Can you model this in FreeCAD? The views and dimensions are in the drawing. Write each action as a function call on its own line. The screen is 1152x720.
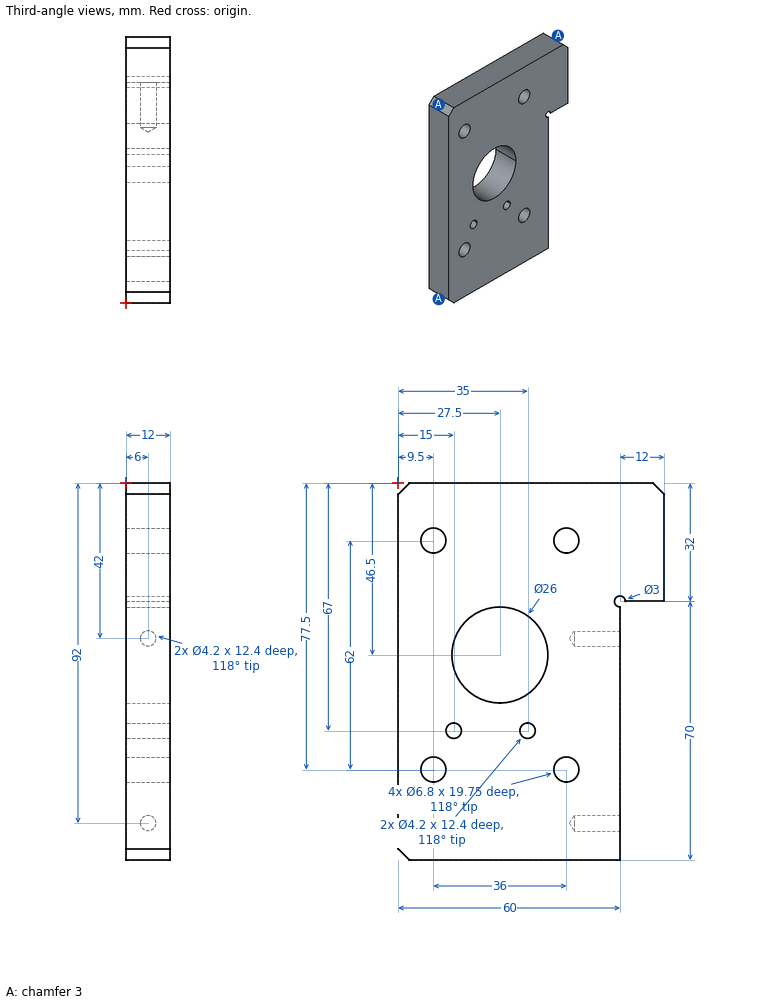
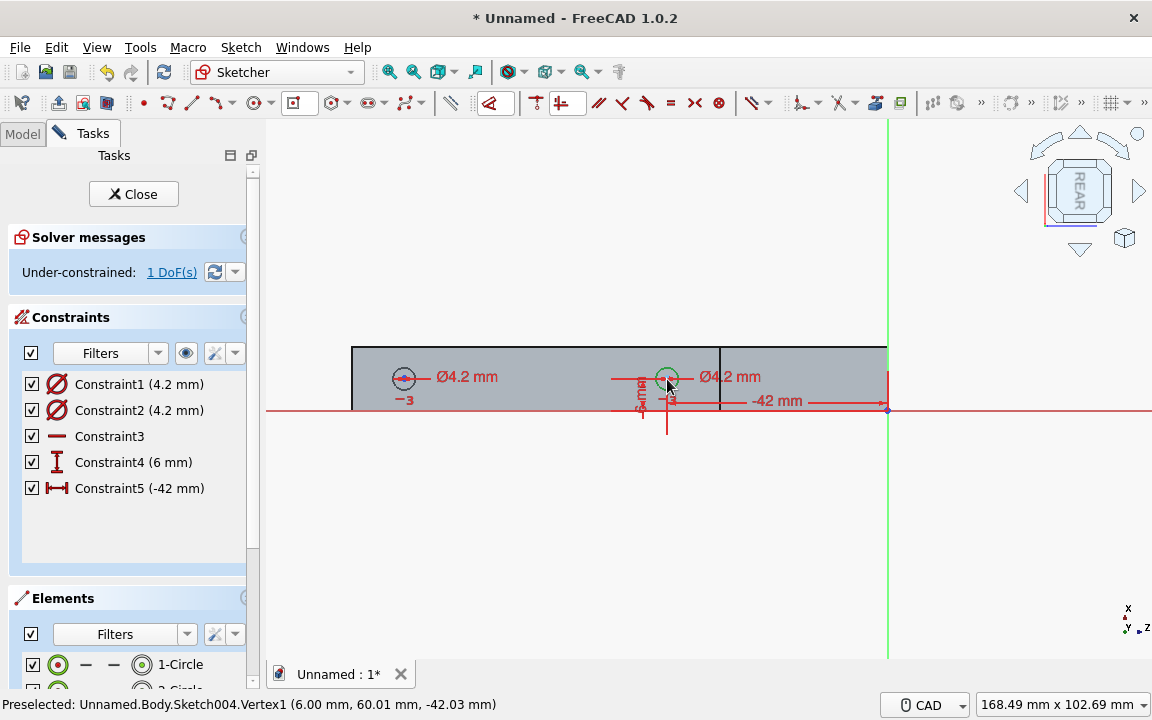
click(404, 379)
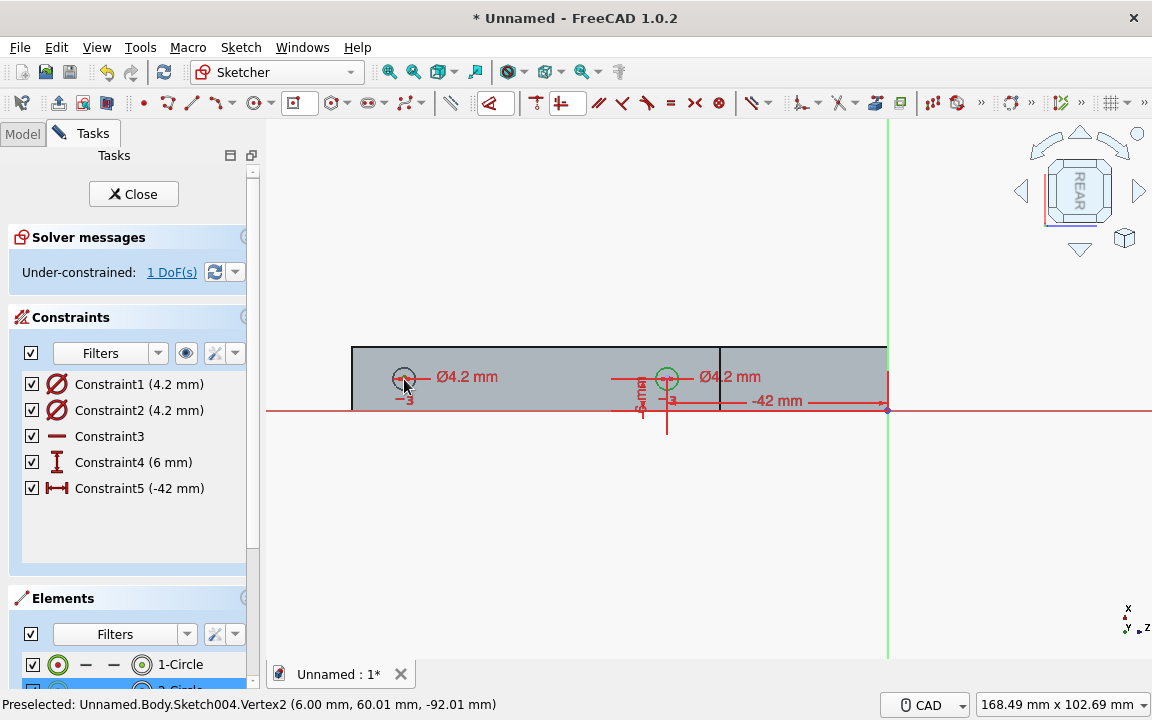
click(508, 104)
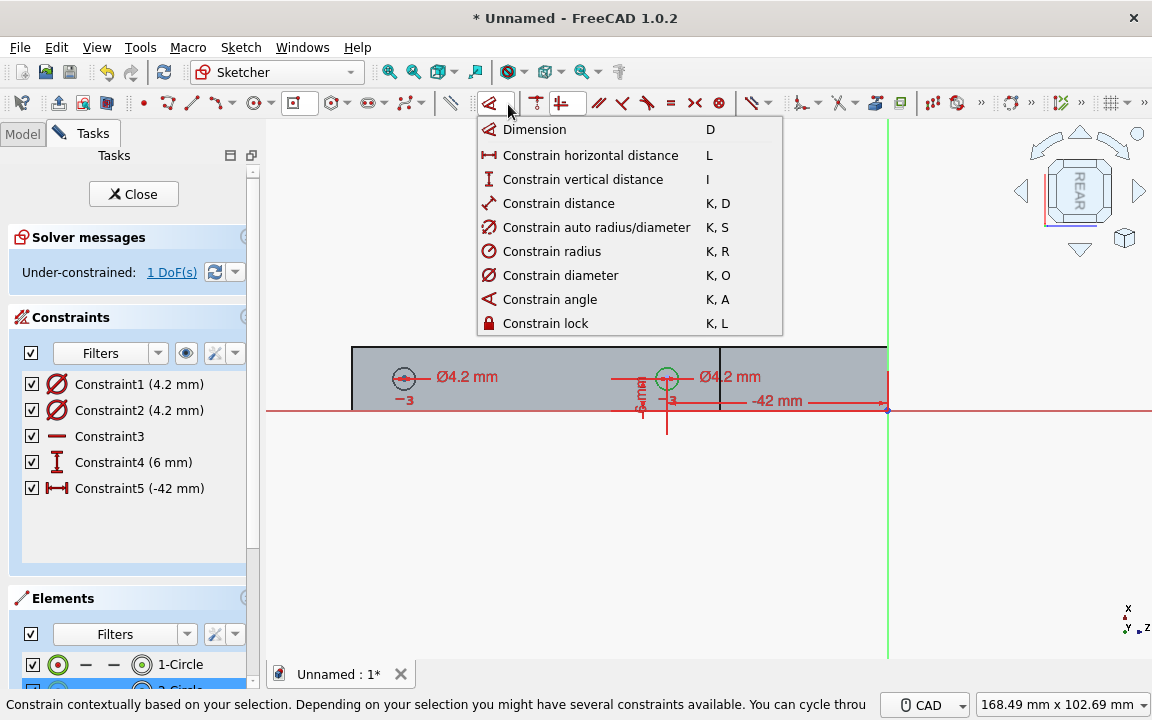
click(630, 155)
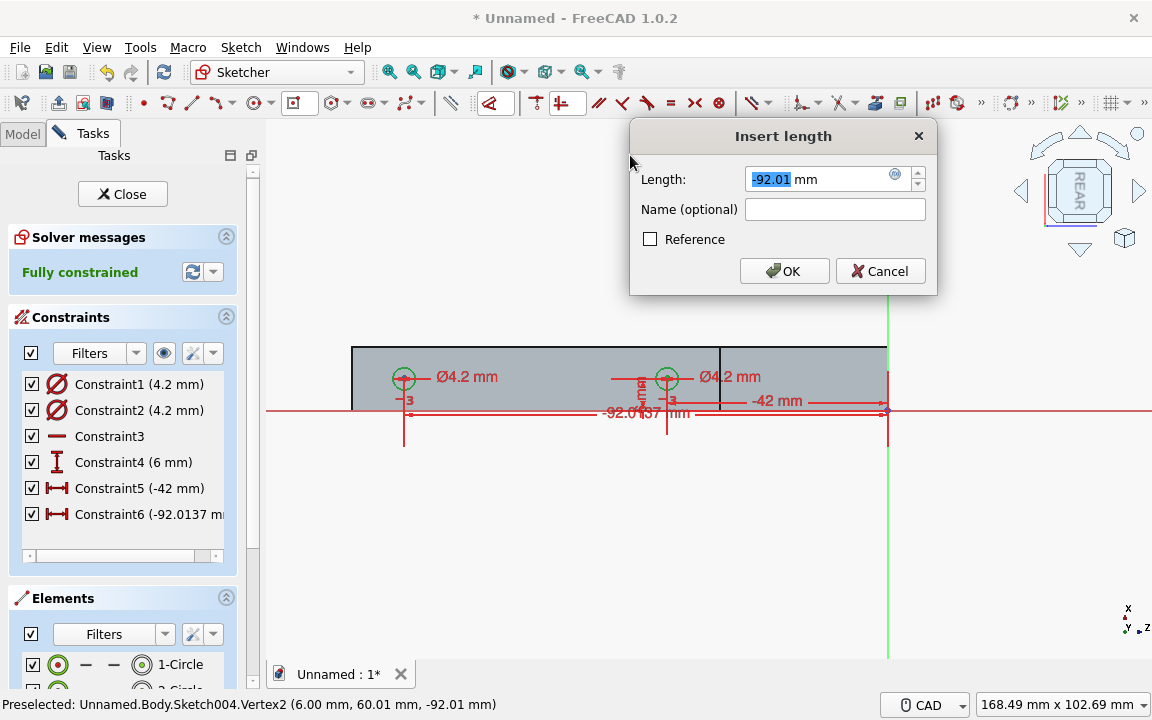
text(-92)
key(Return)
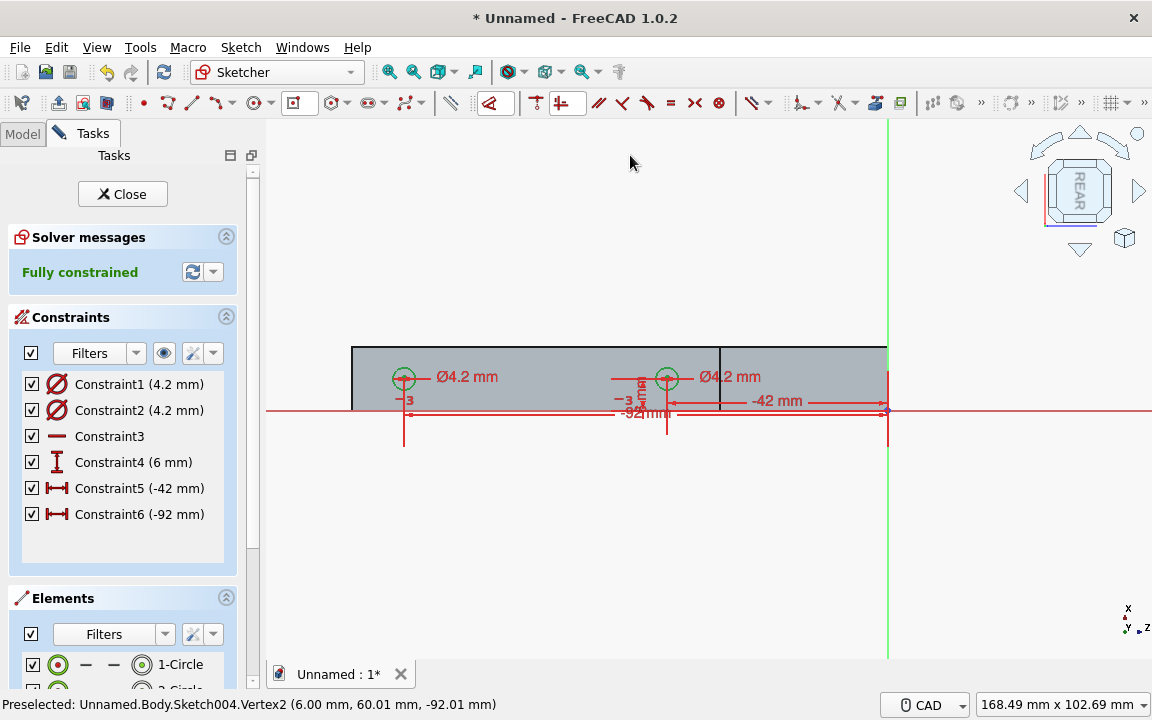
click(123, 194)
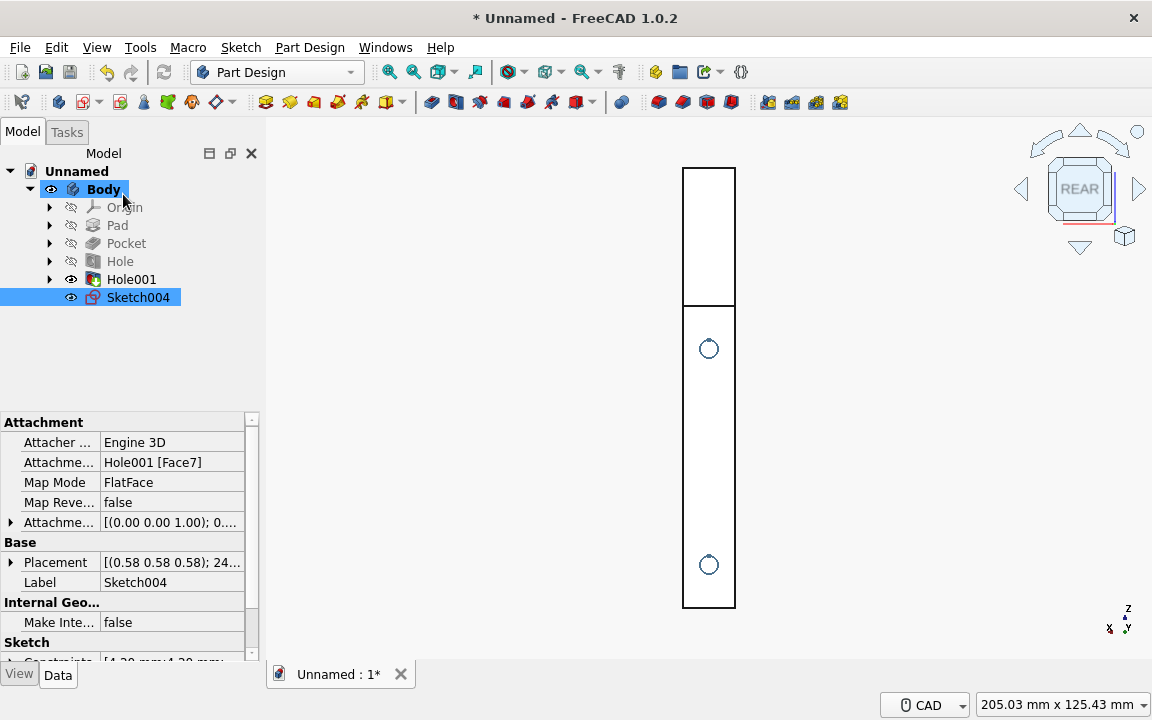
click(456, 102)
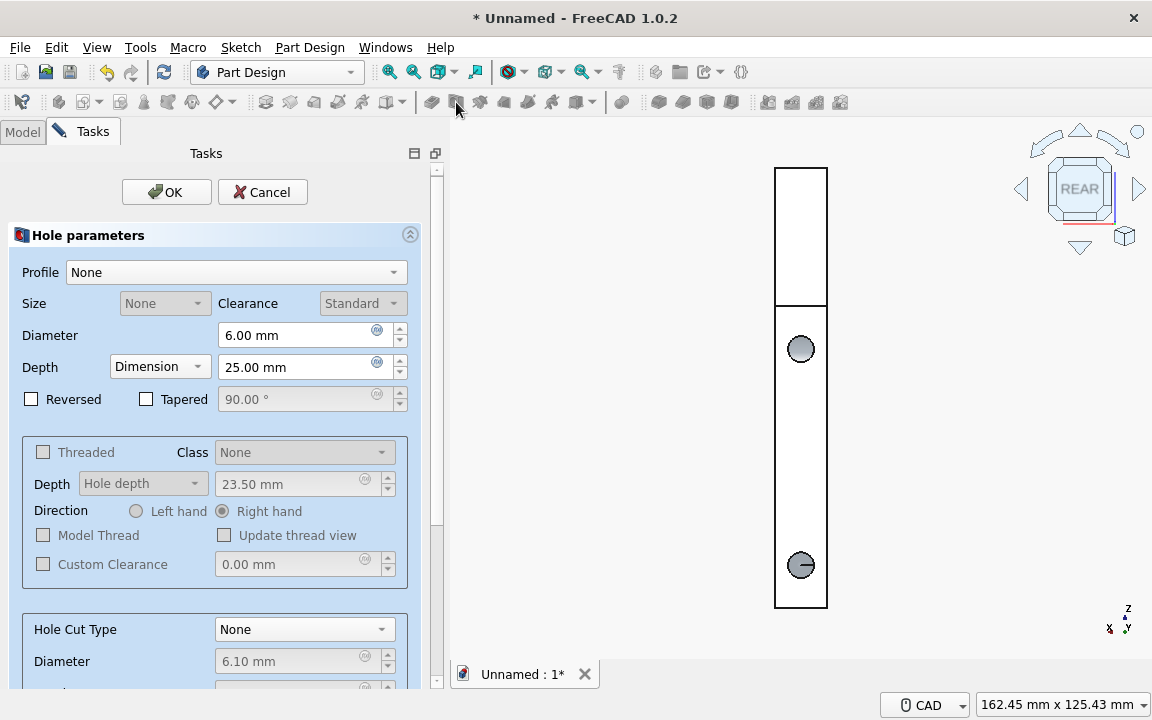
triple_click(305, 335)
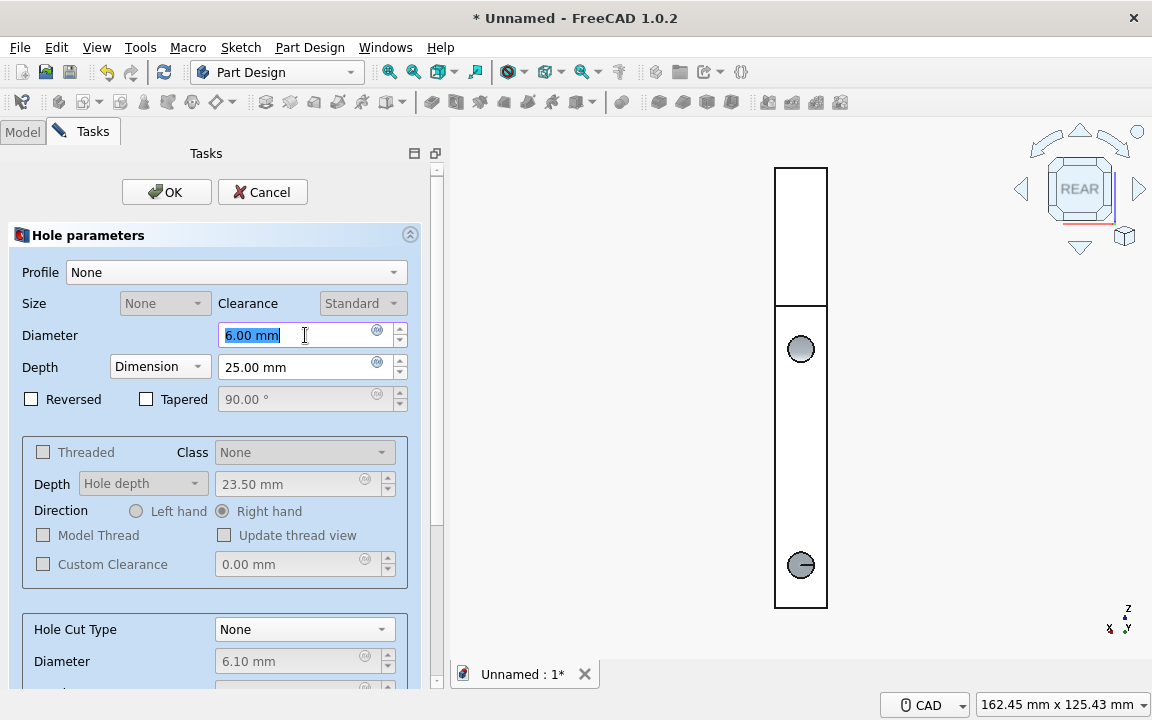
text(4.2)
key(Tab)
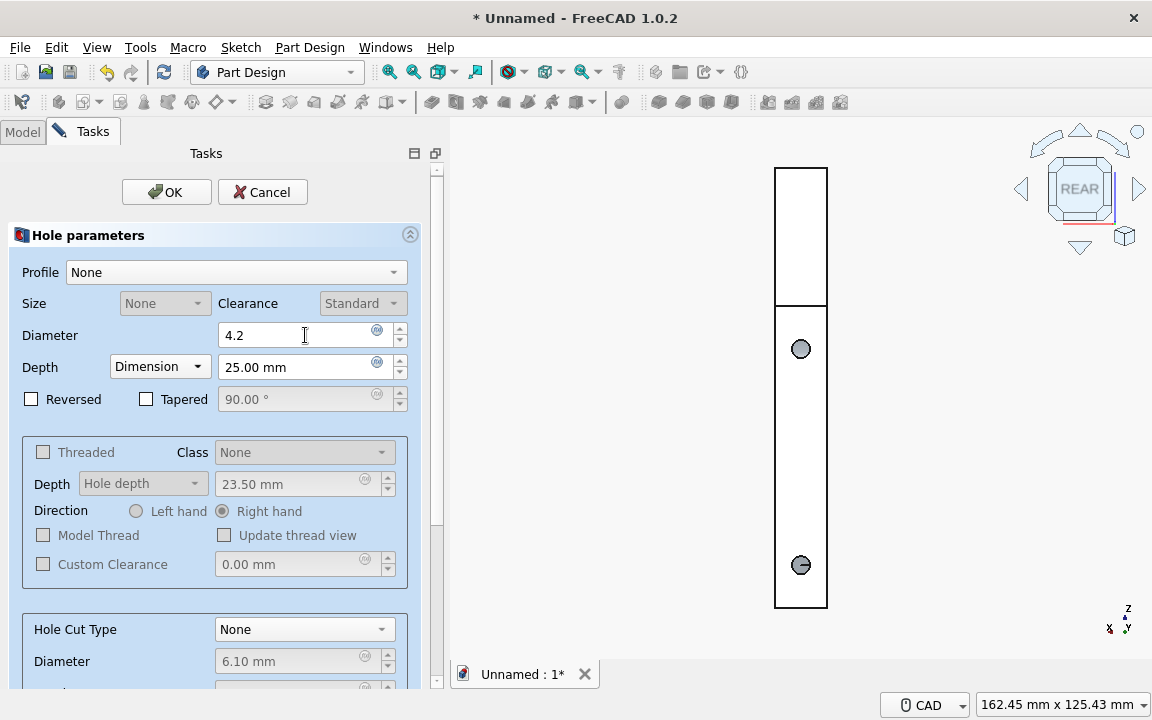
triple_click(305, 367)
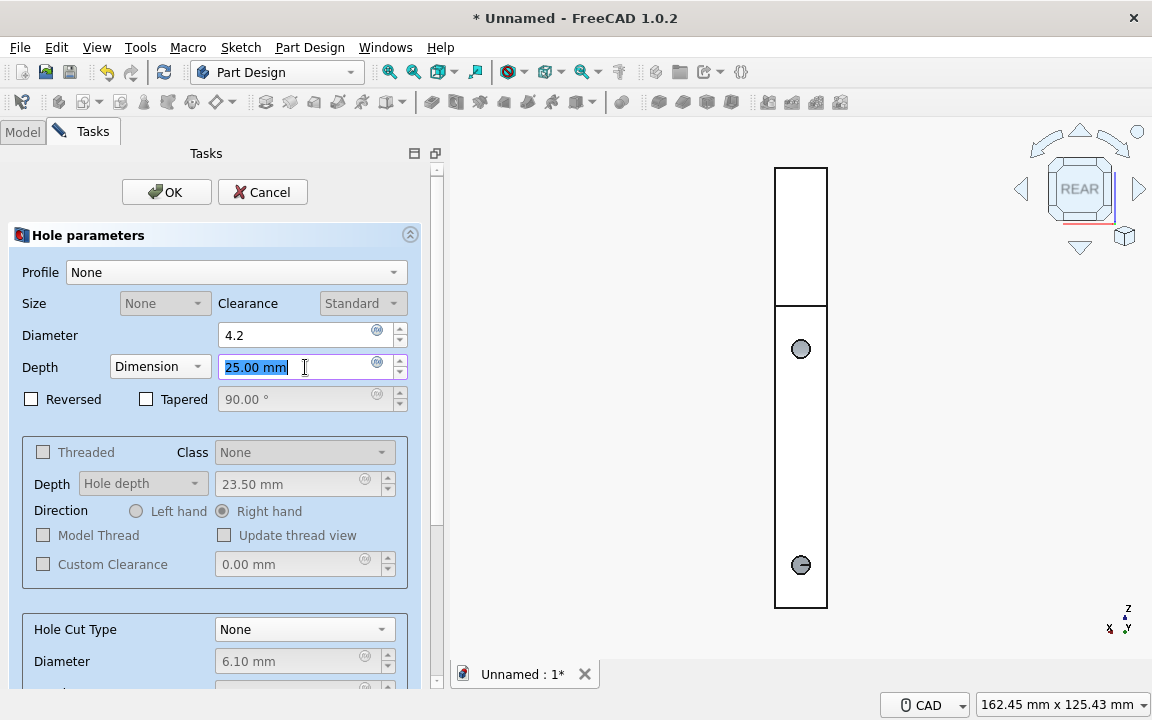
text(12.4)
key(Tab)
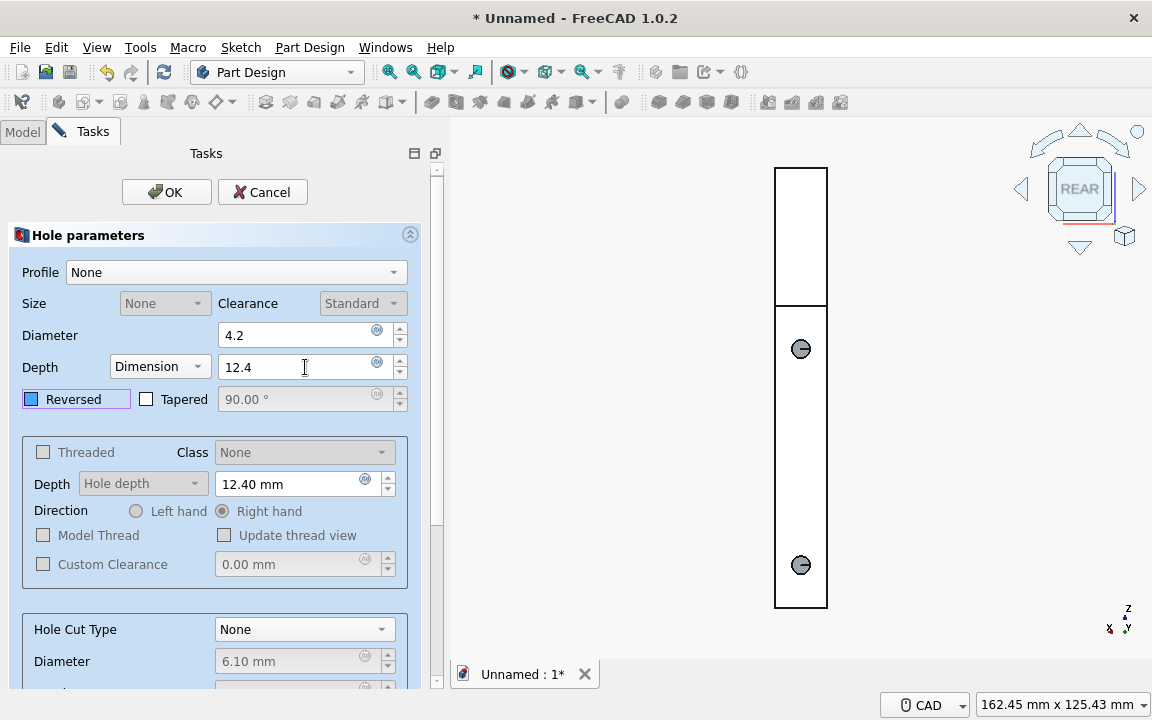
click(167, 192)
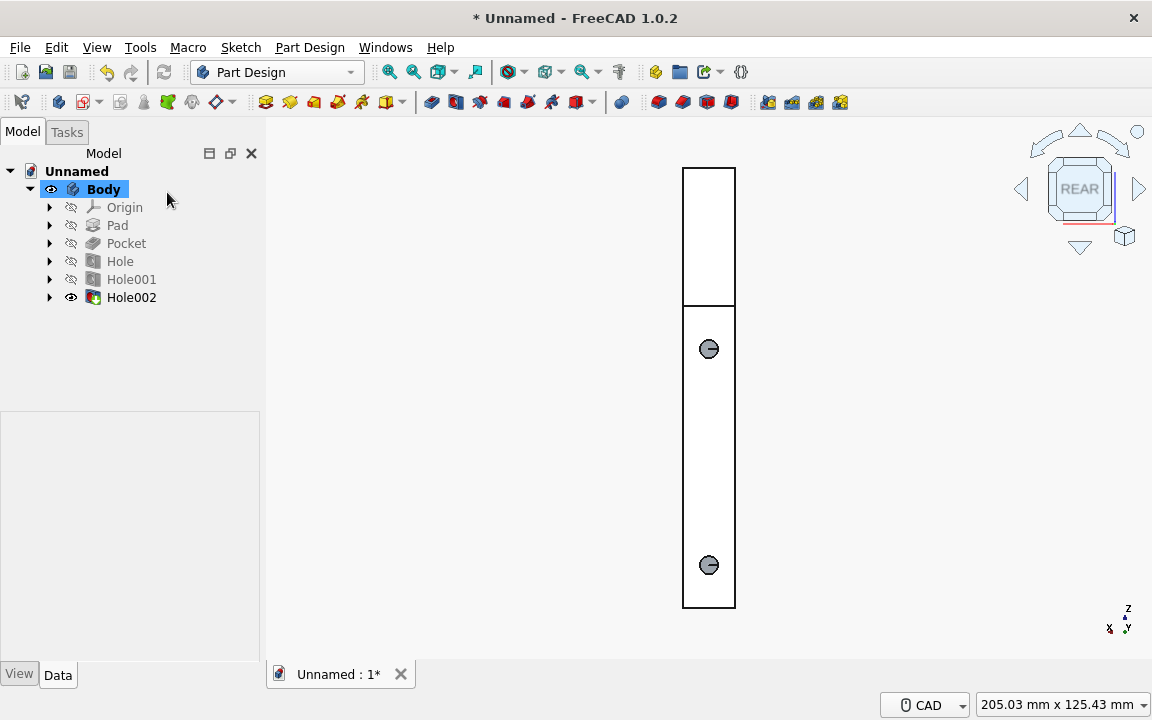
click(709, 167)